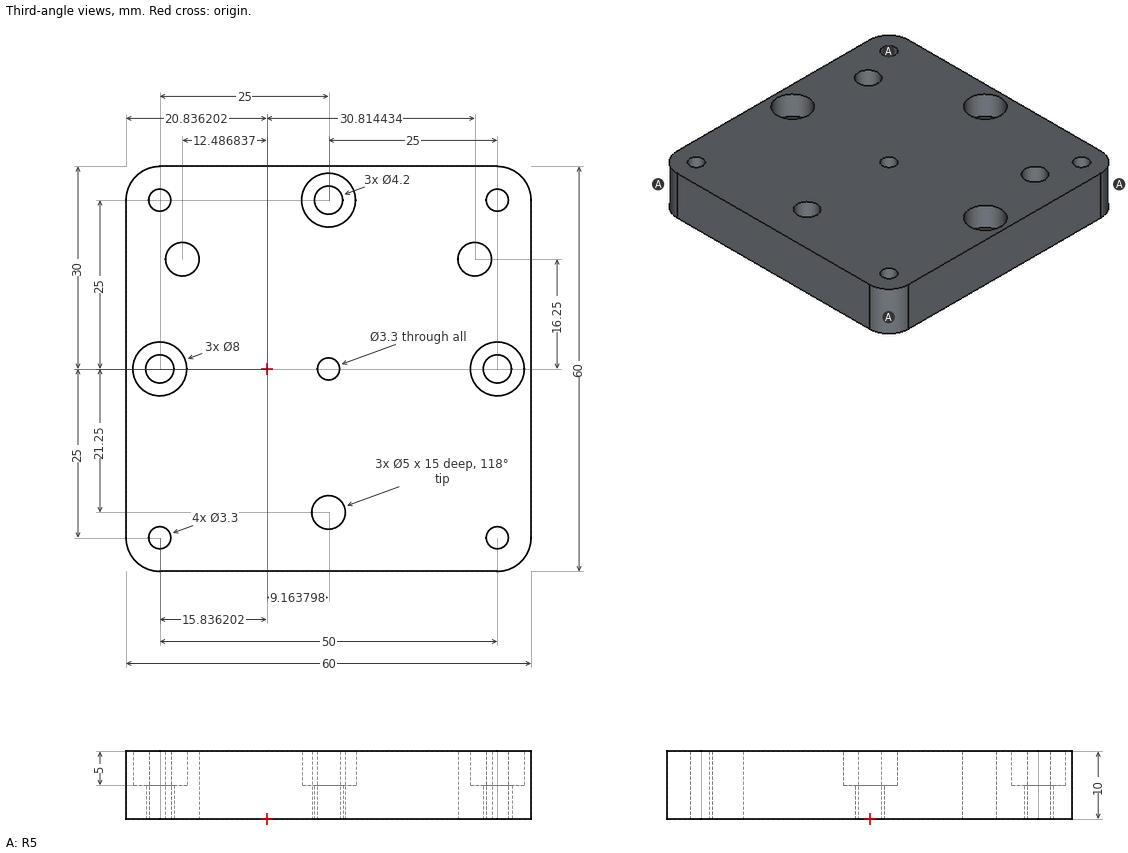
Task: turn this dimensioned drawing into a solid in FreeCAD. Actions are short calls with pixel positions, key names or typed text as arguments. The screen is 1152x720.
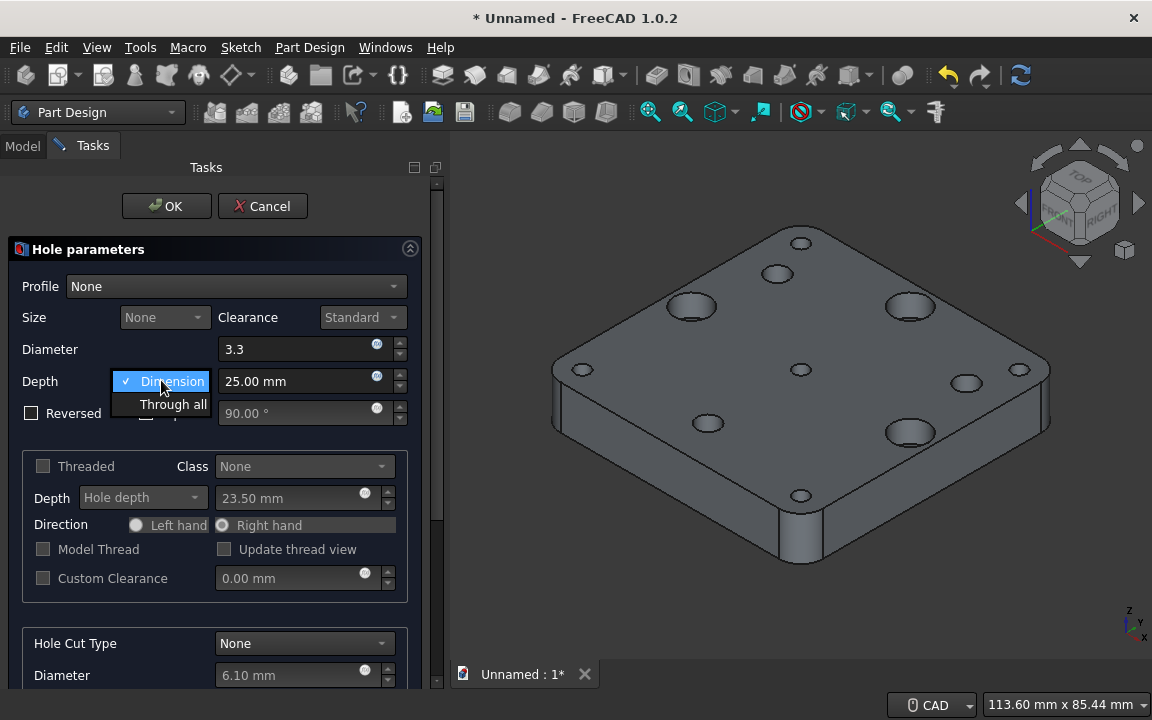
click(160, 404)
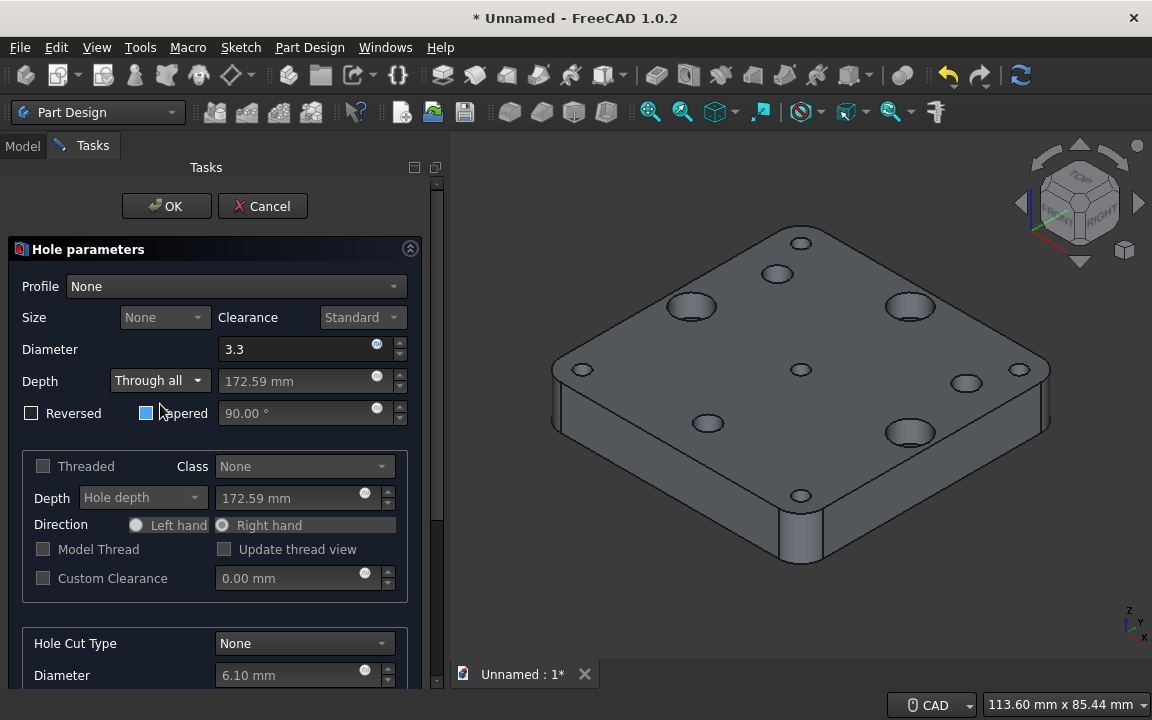
click(167, 206)